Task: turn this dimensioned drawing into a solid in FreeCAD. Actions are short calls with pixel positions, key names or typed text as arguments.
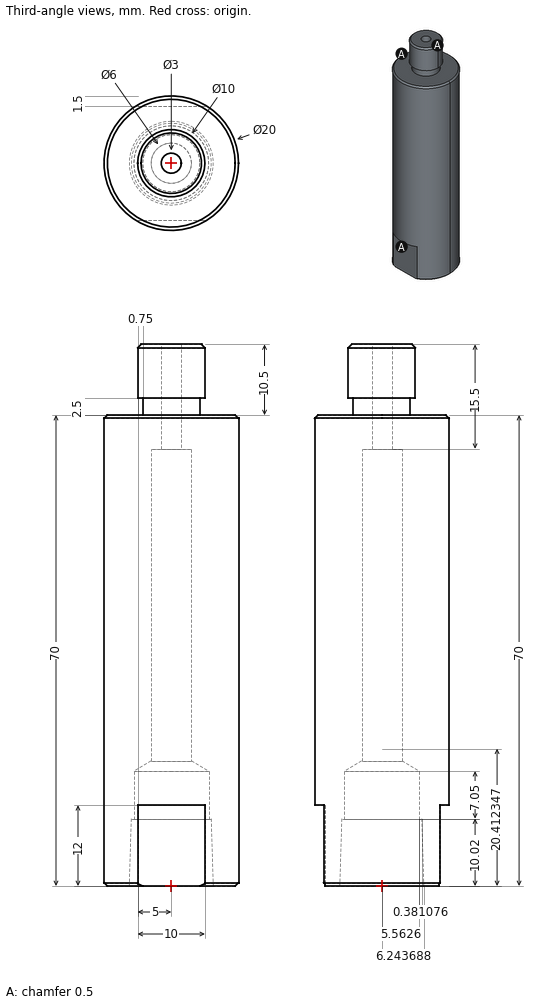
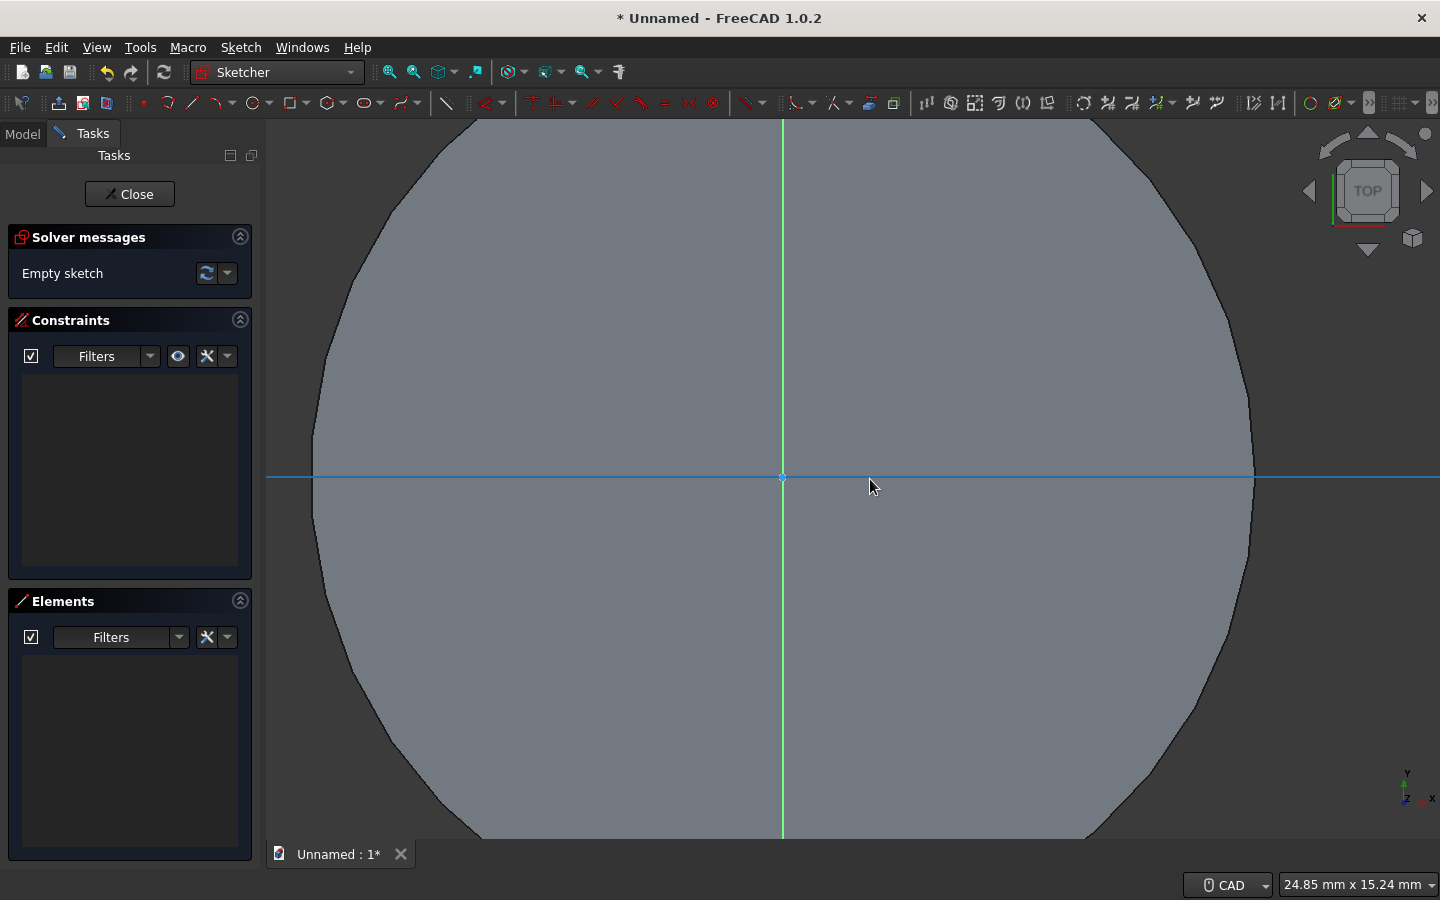
key(g)
key(c)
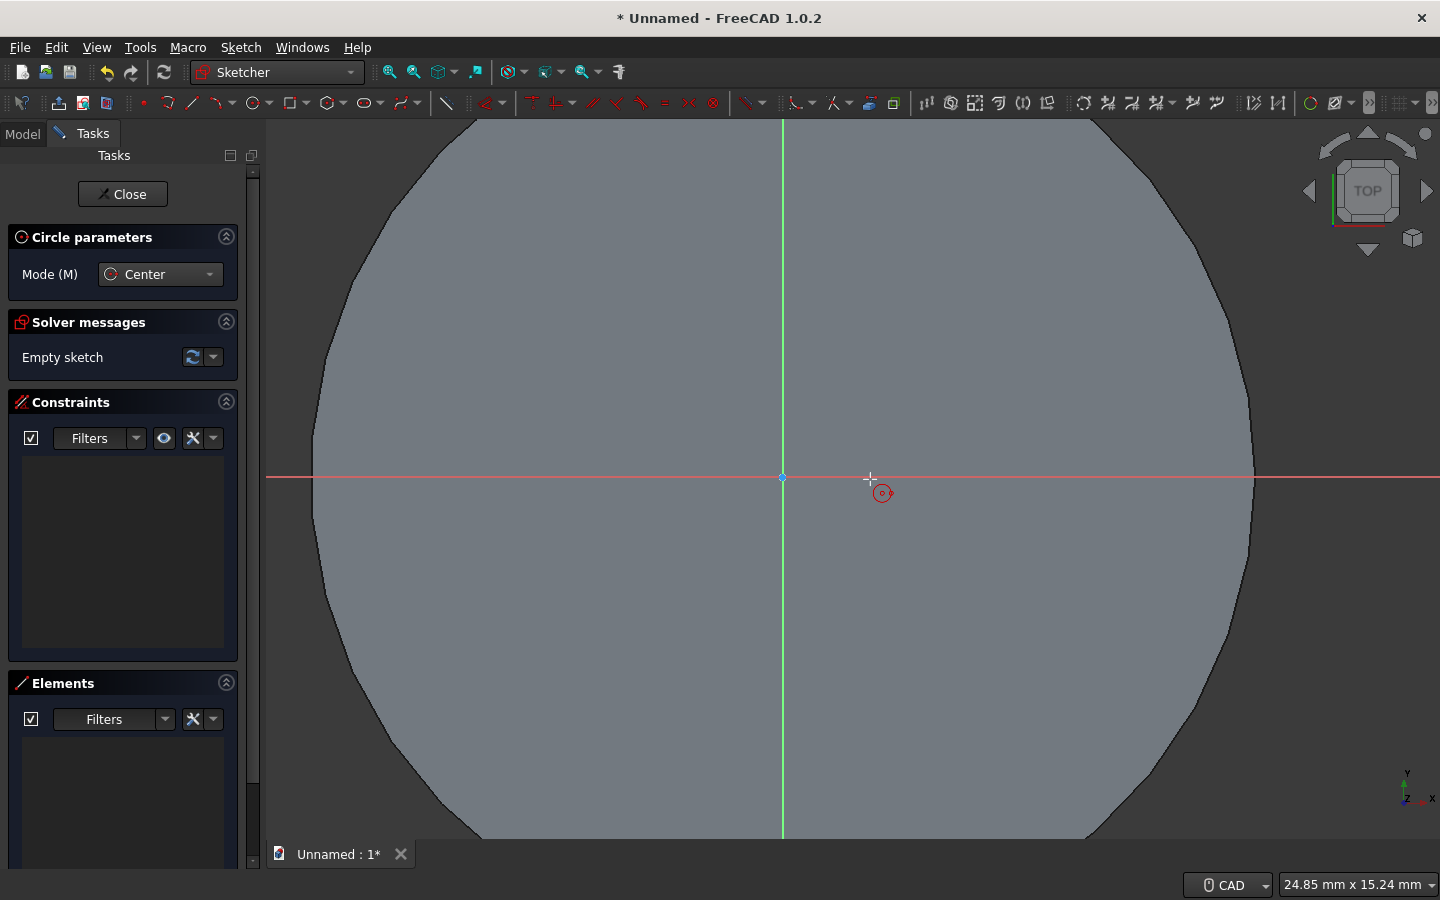
click(783, 477)
move(950, 310)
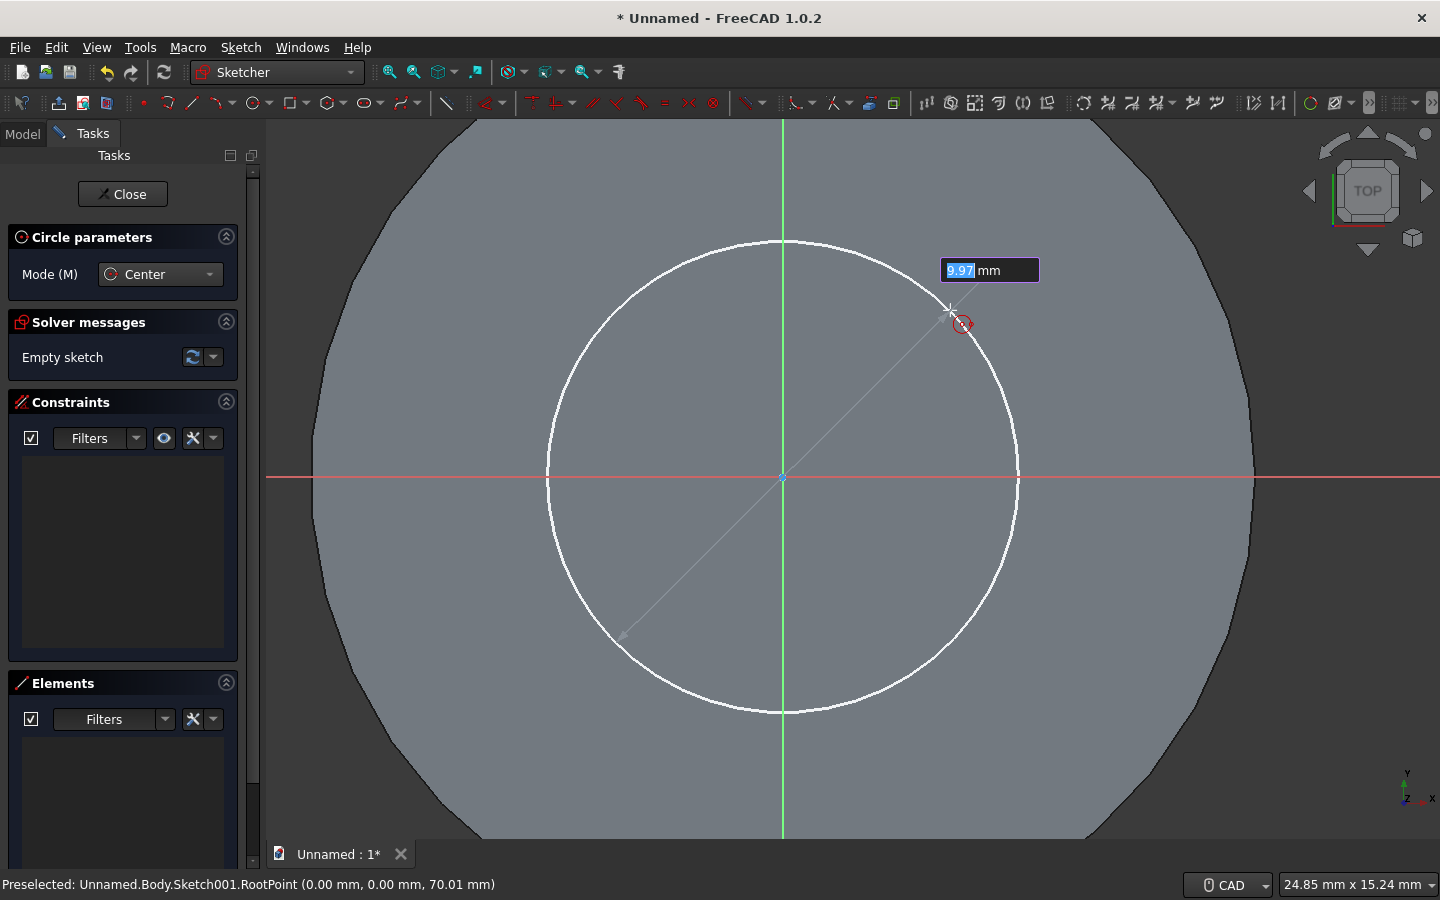
text(10)
key(Return)
key(Escape)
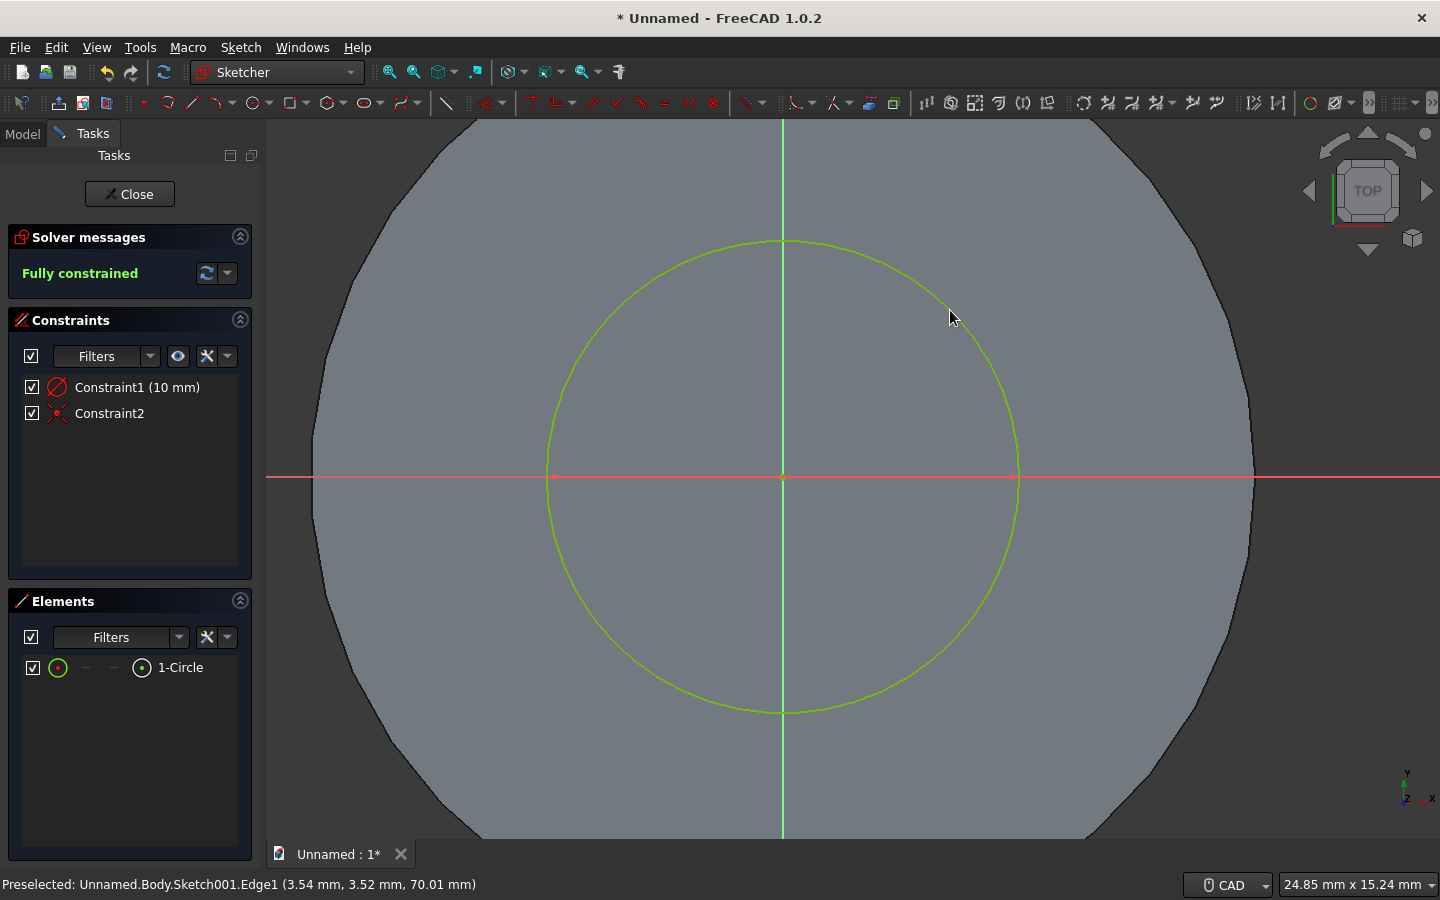
click(130, 194)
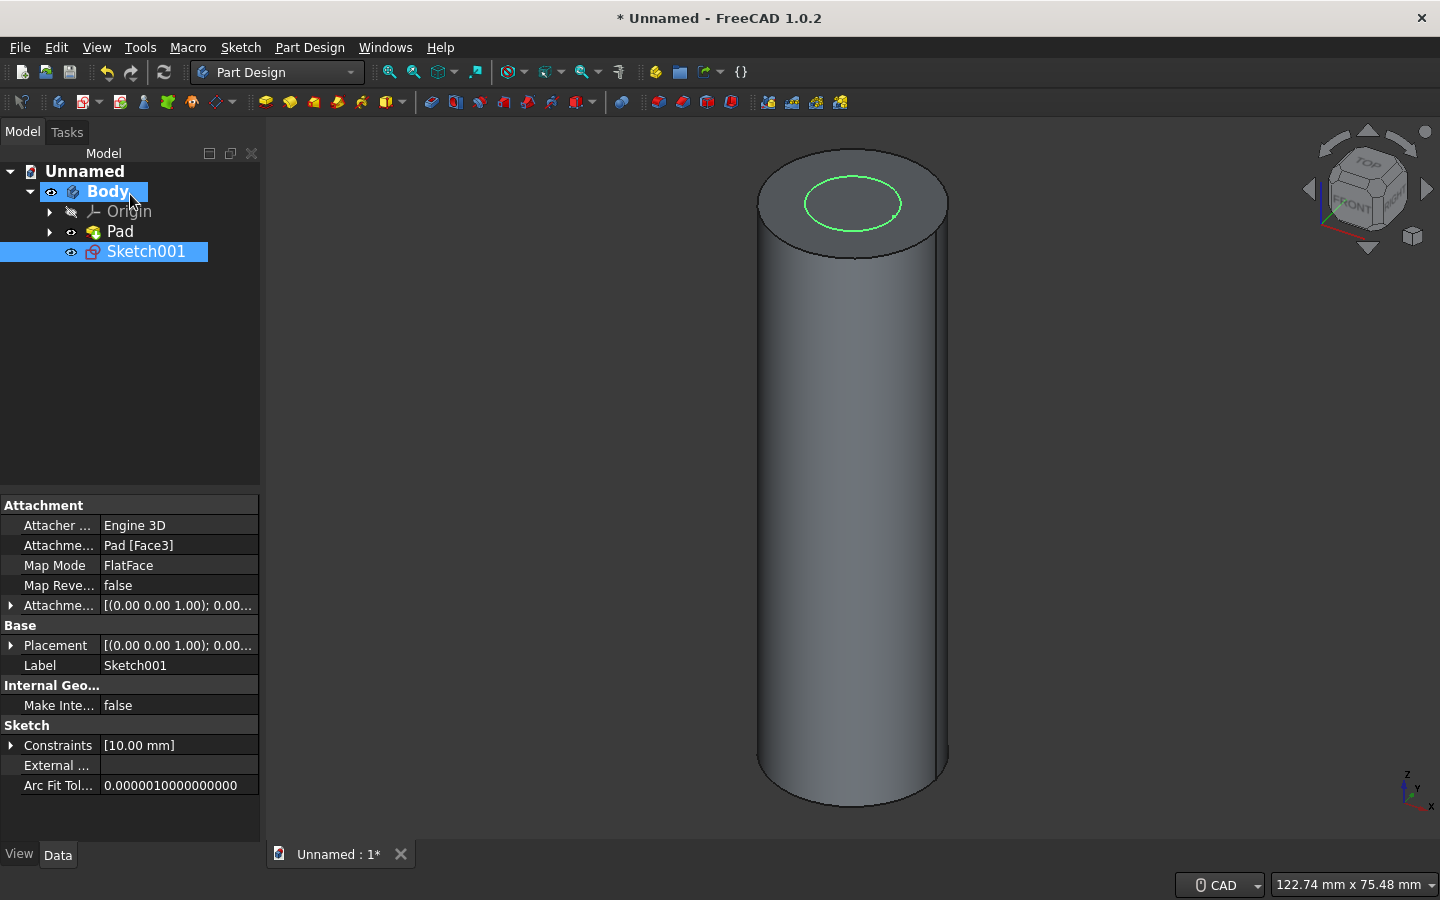
click(266, 102)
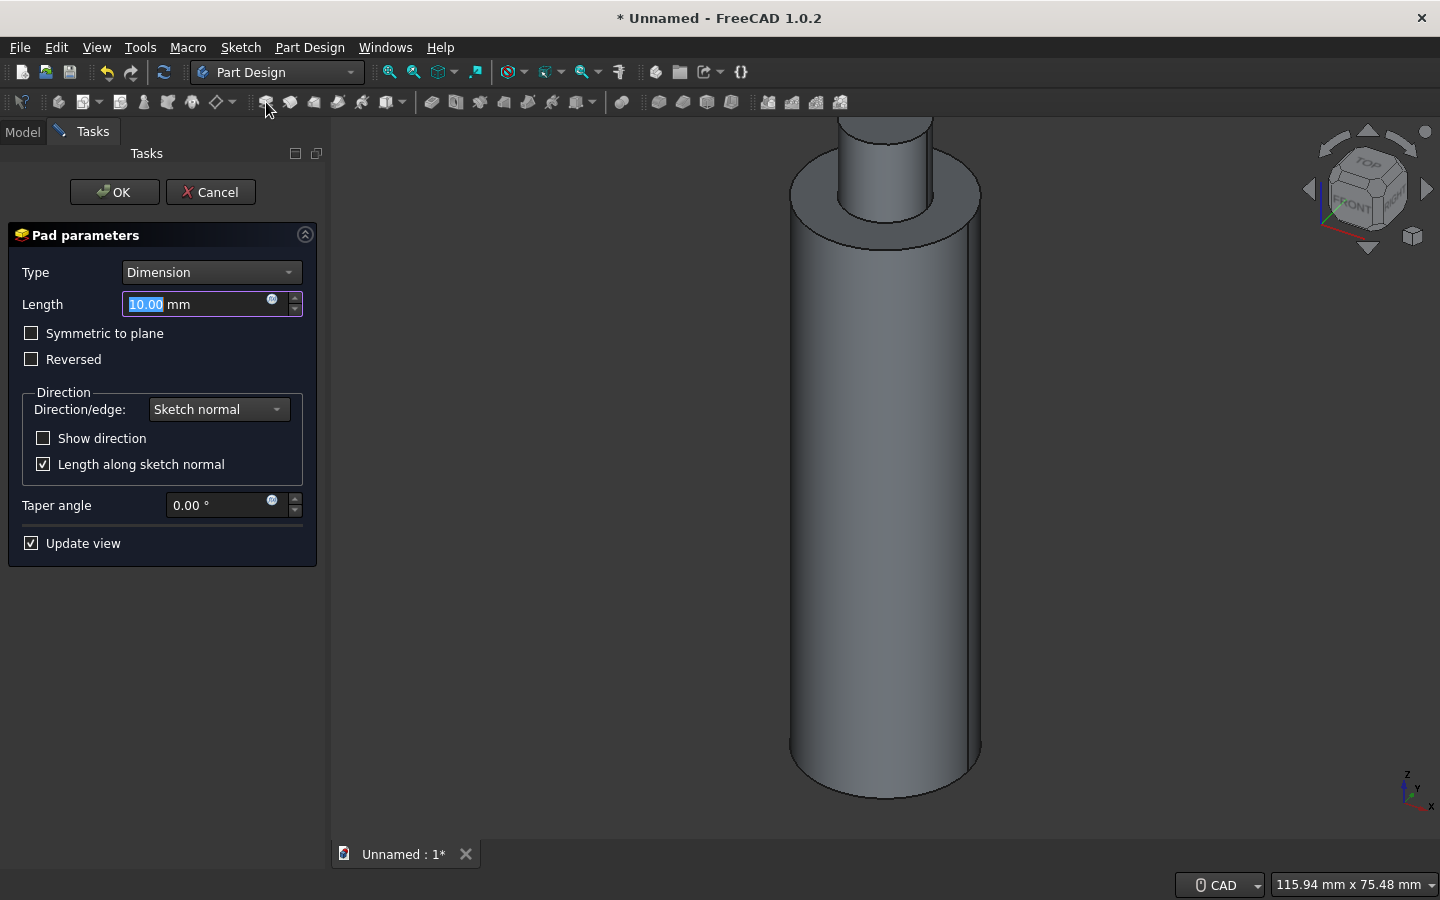
text(10.5)
key(Tab)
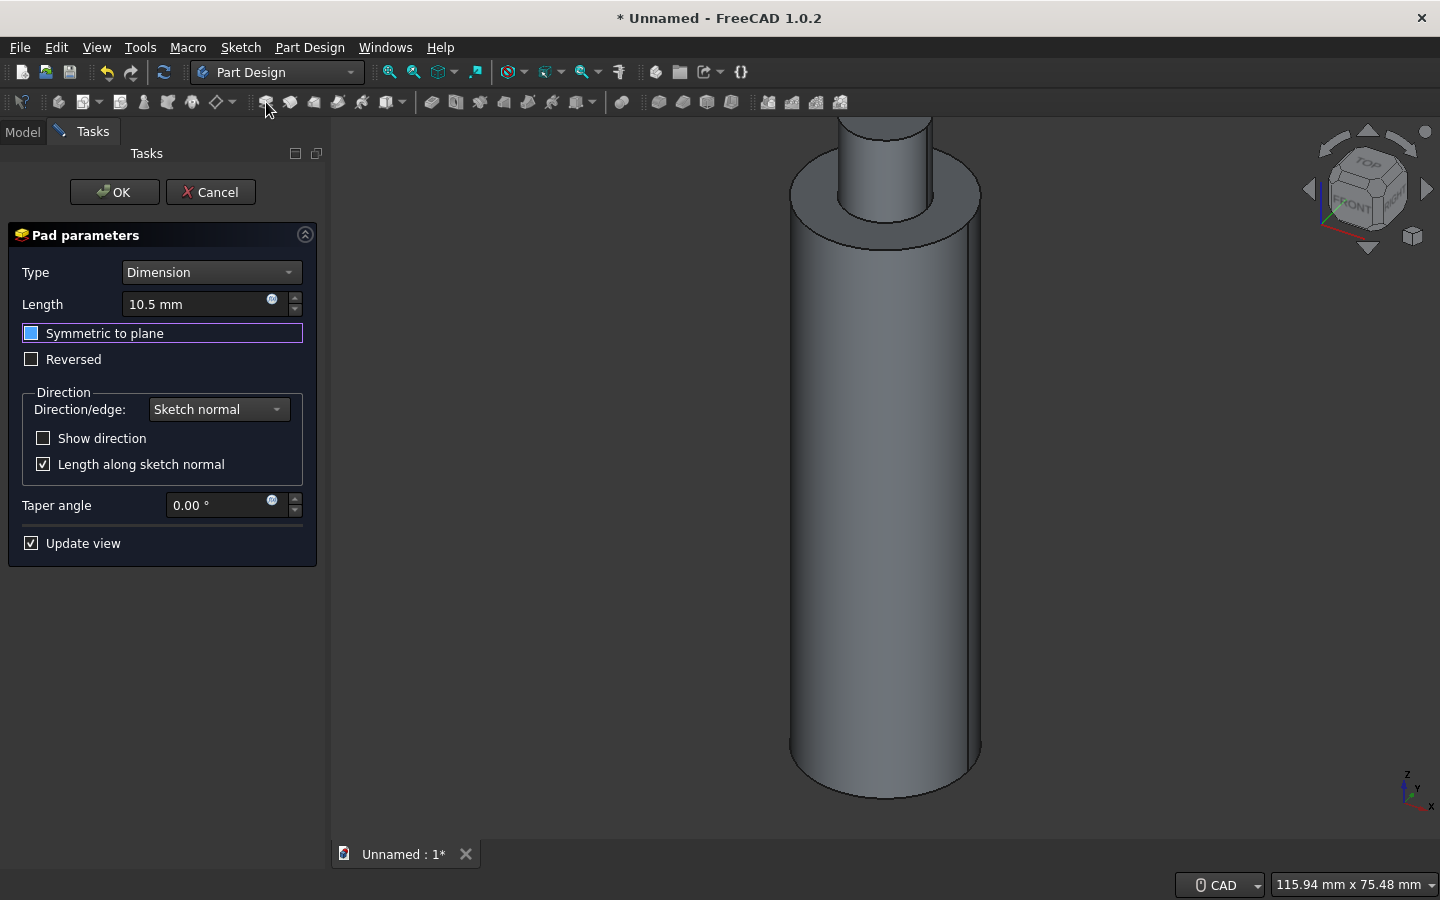
click(115, 192)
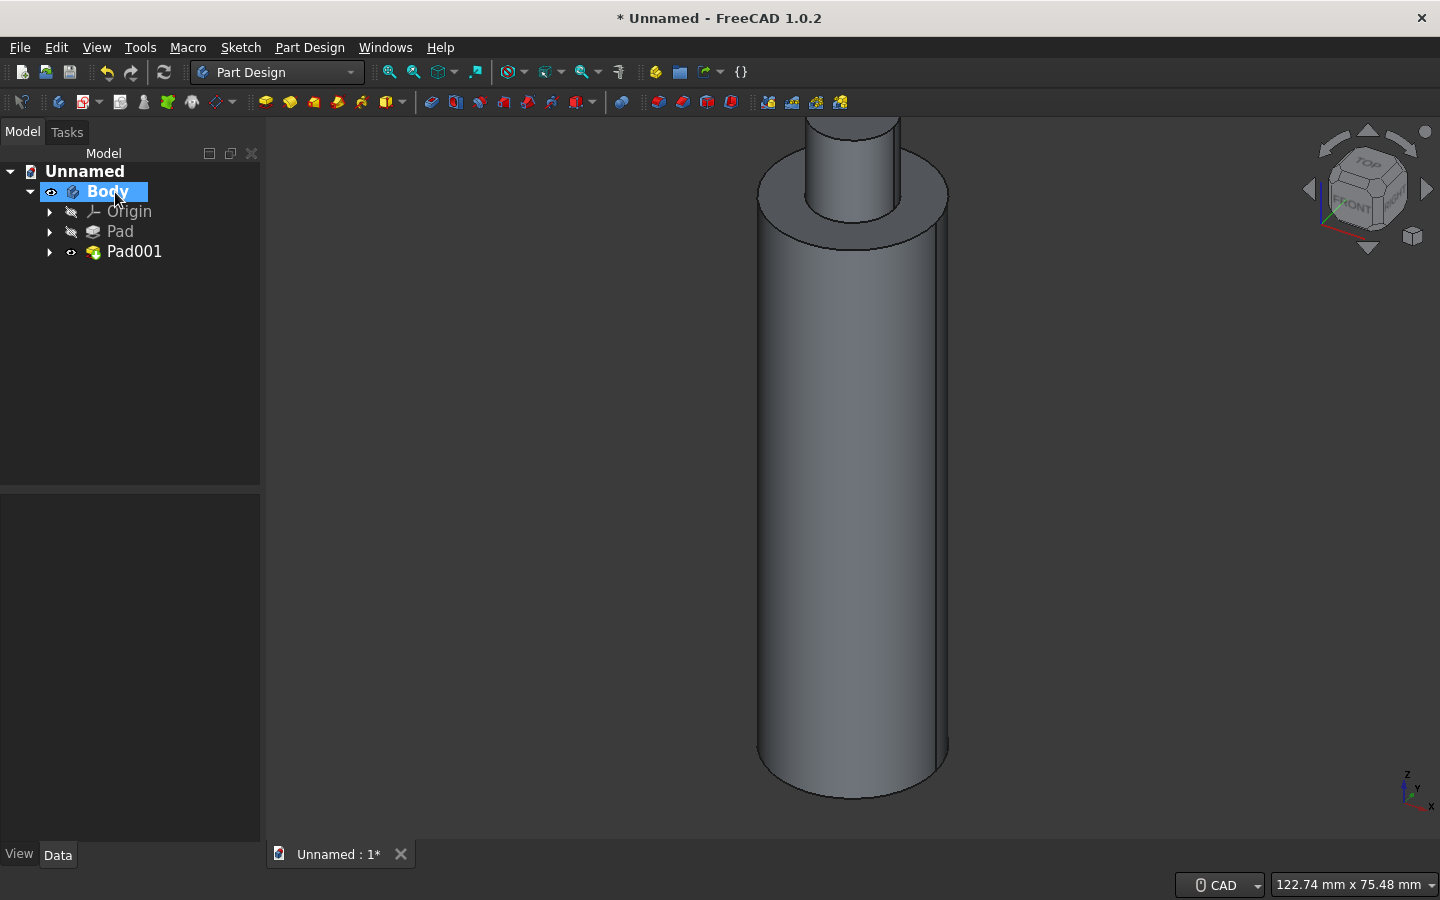
click(390, 72)